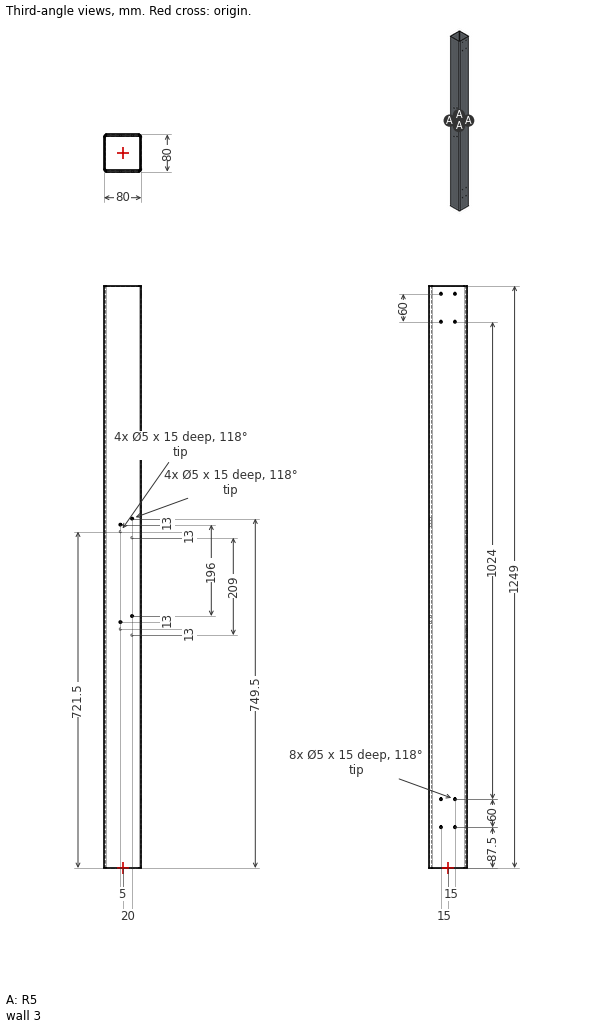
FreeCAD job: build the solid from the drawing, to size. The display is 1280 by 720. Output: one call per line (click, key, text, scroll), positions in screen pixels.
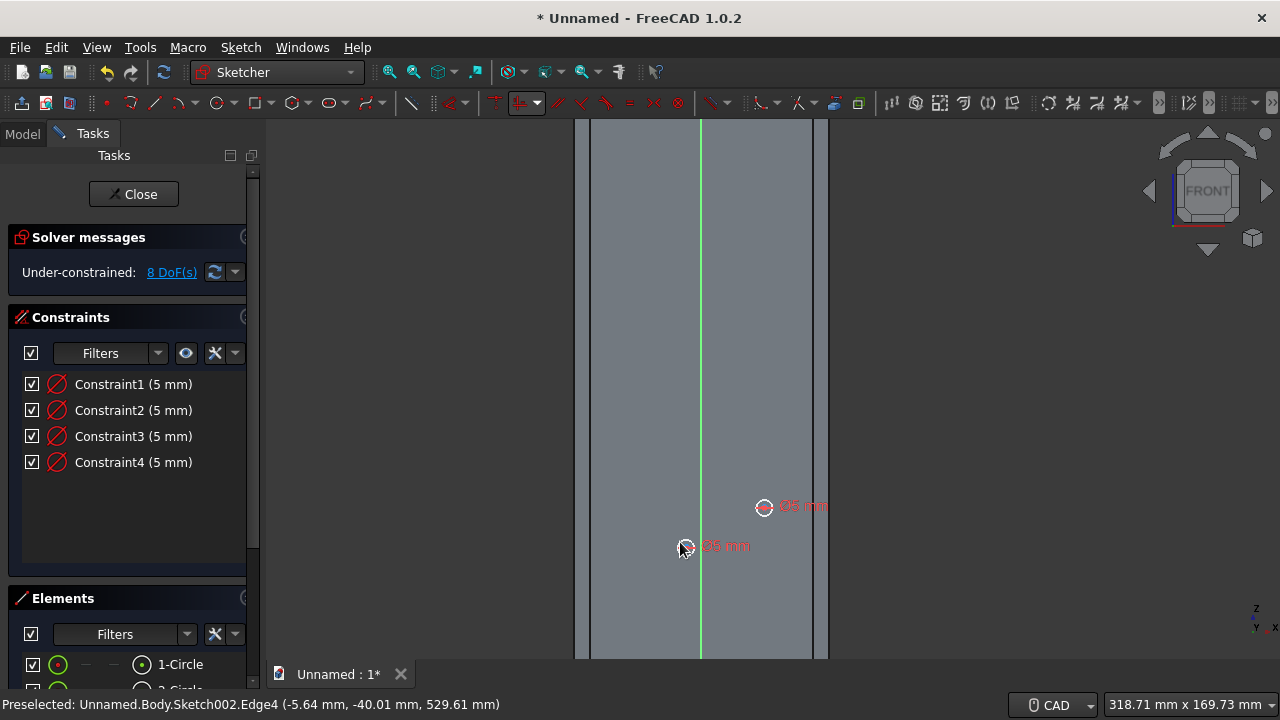
scroll(687, 548, down, 4)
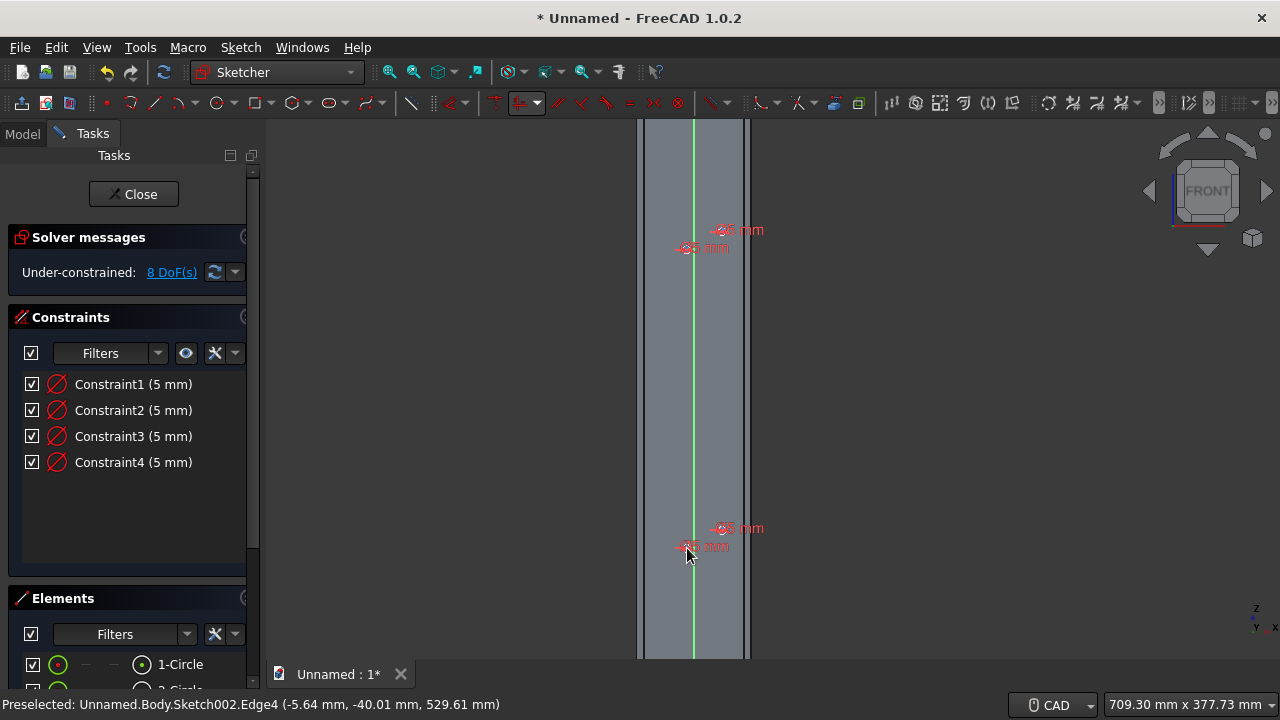
click(722, 232)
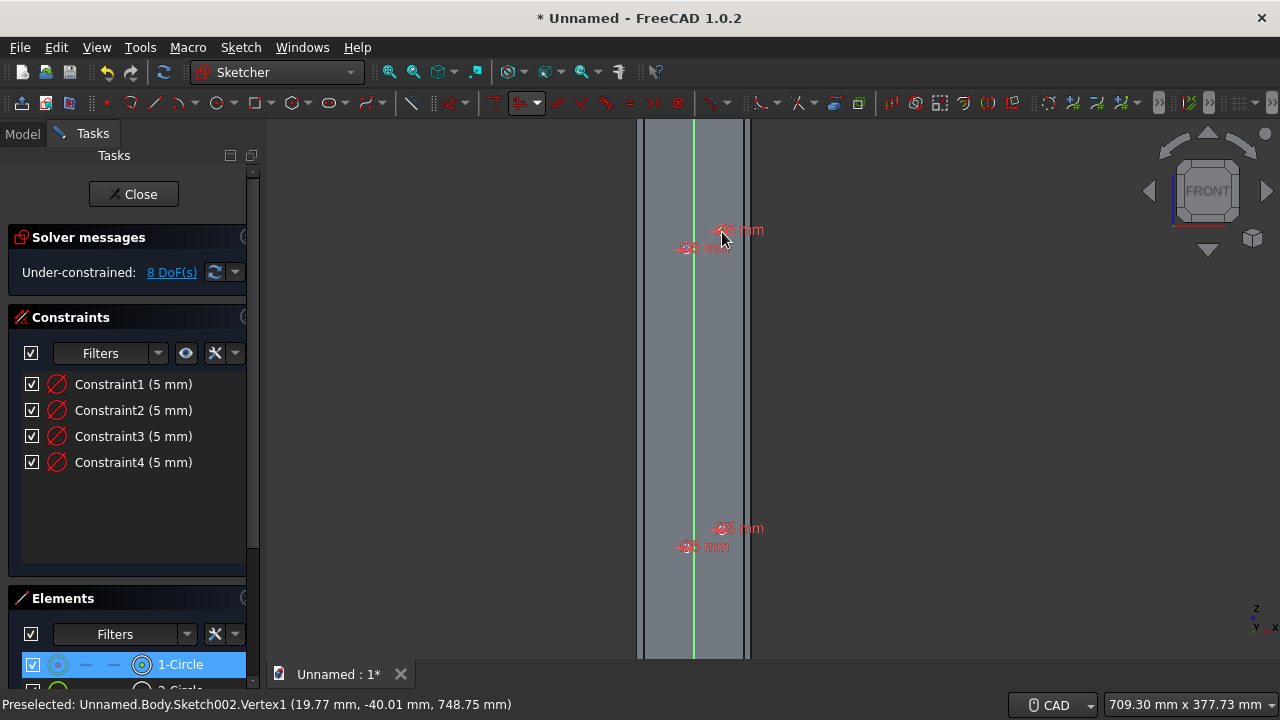
click(722, 530)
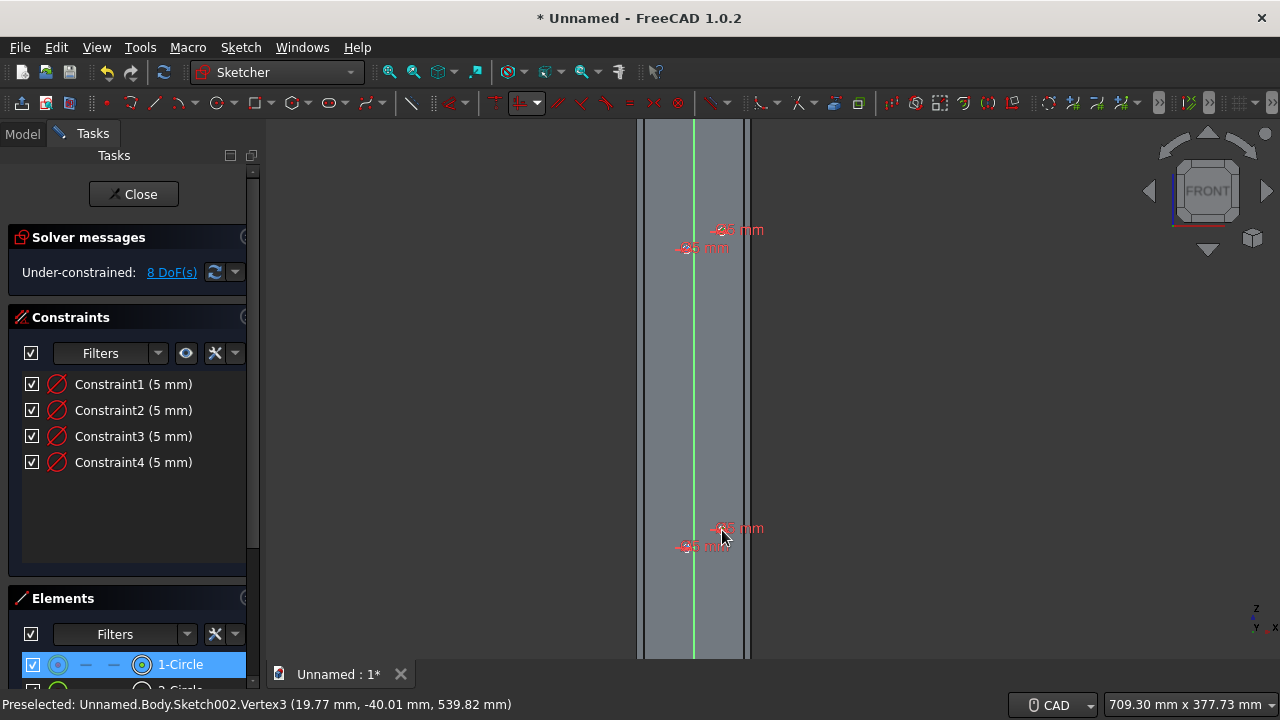
key(v)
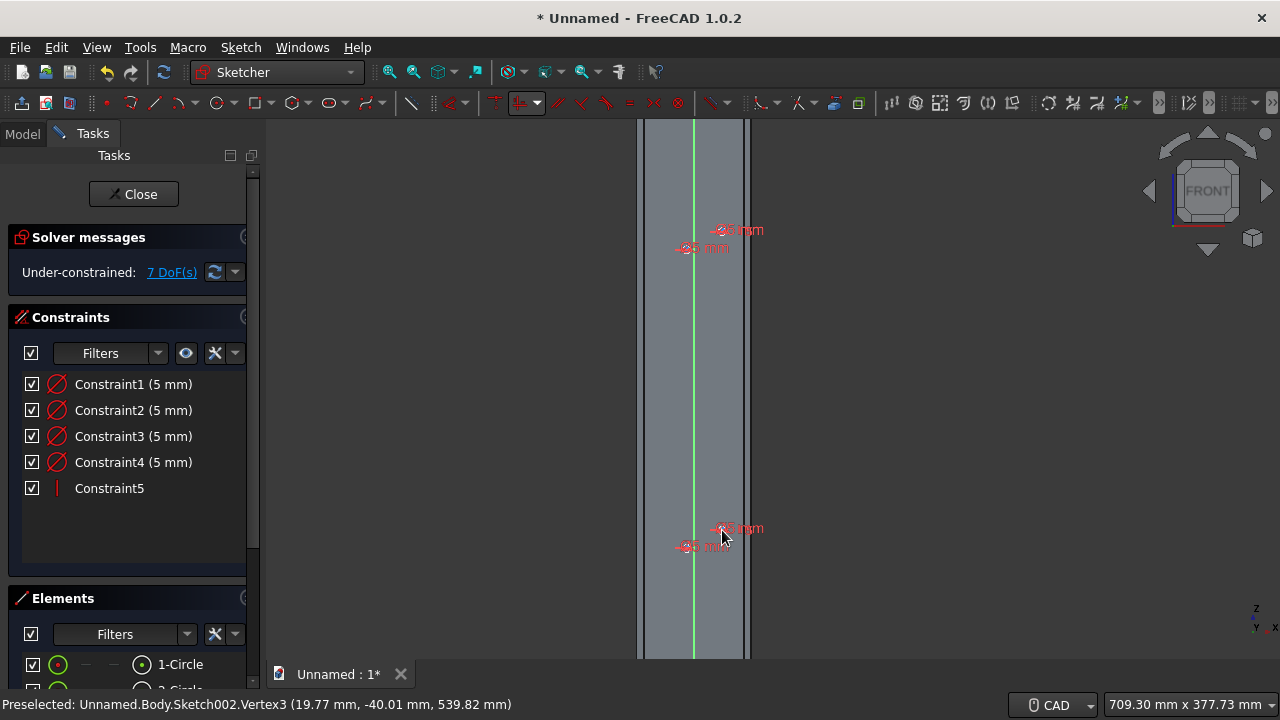
click(687, 250)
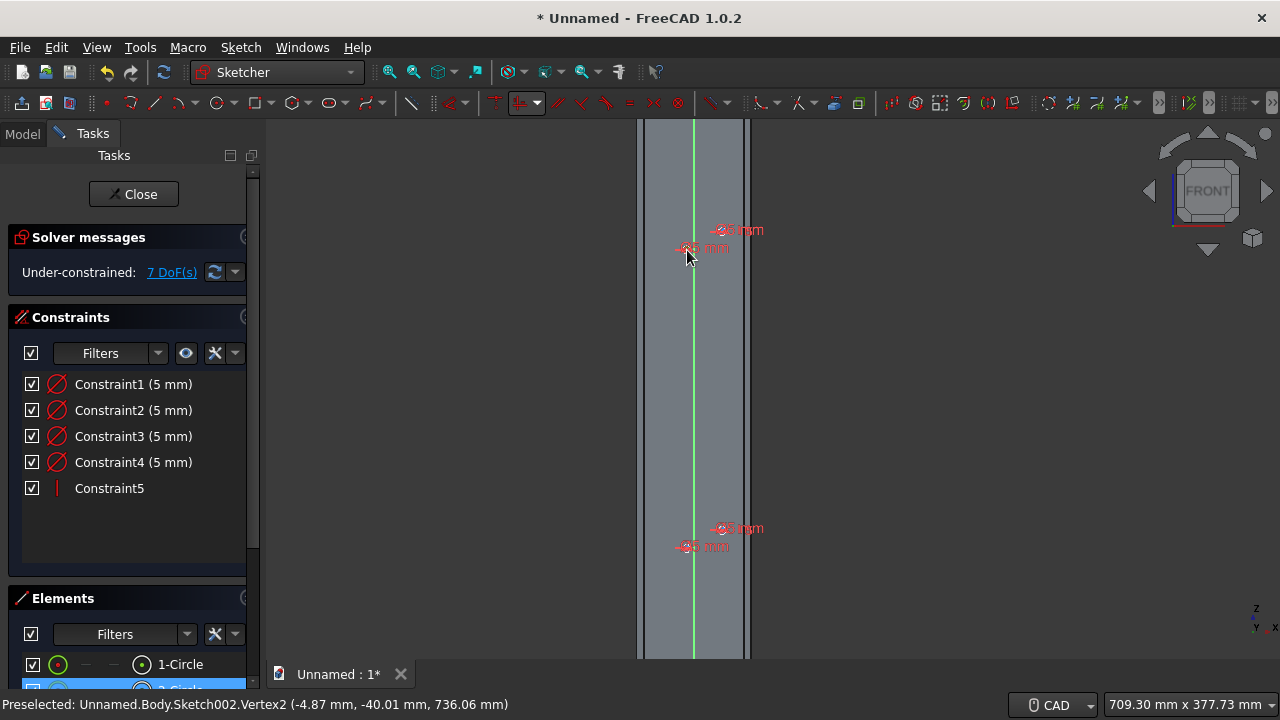
click(687, 548)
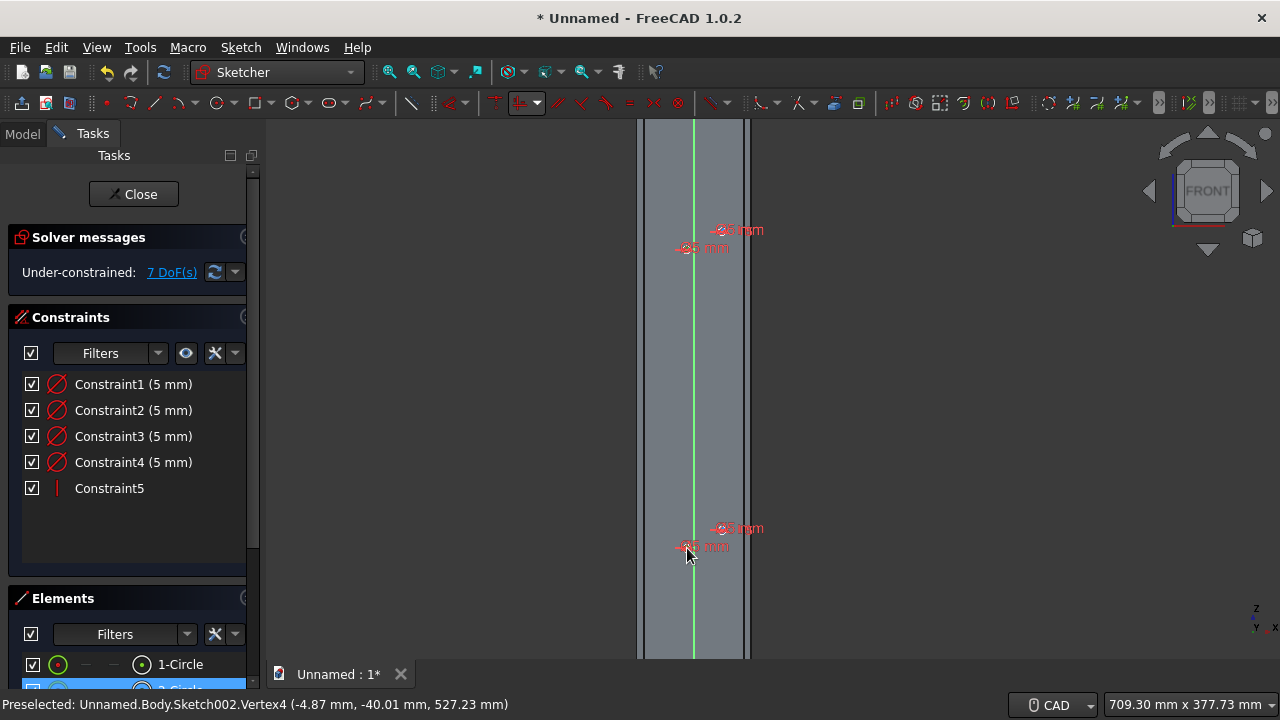
key(v)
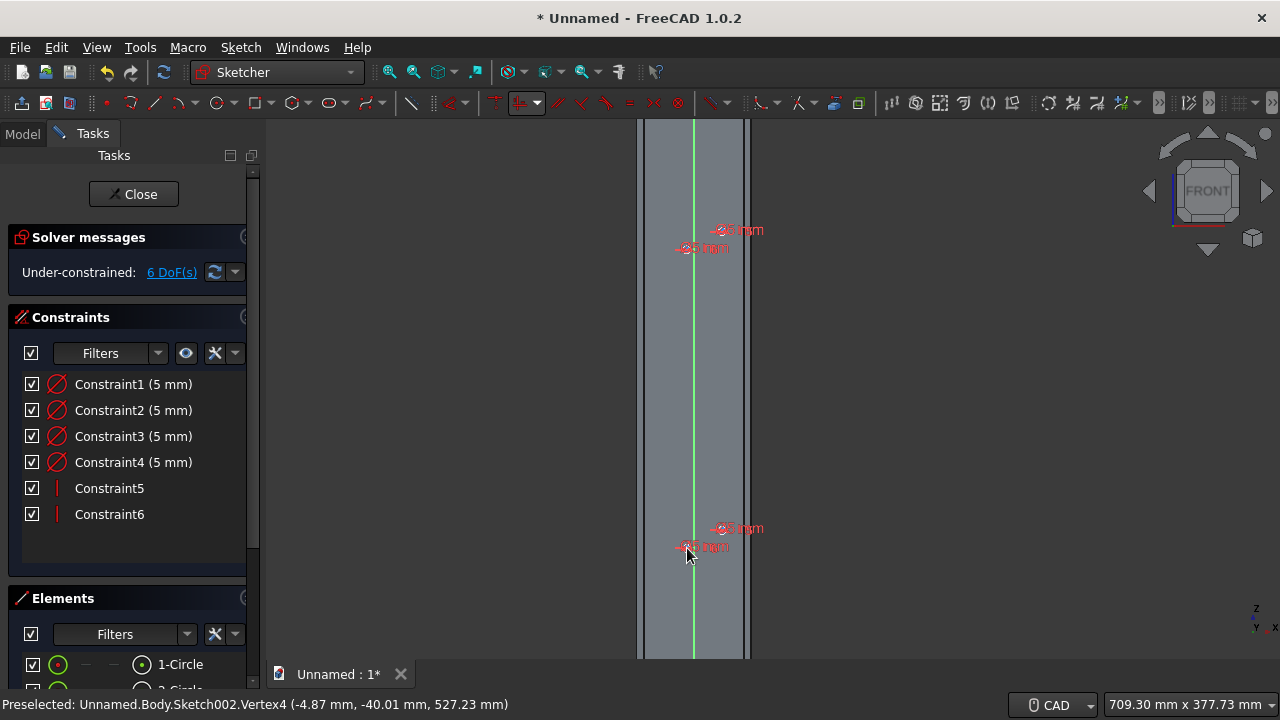
key(d)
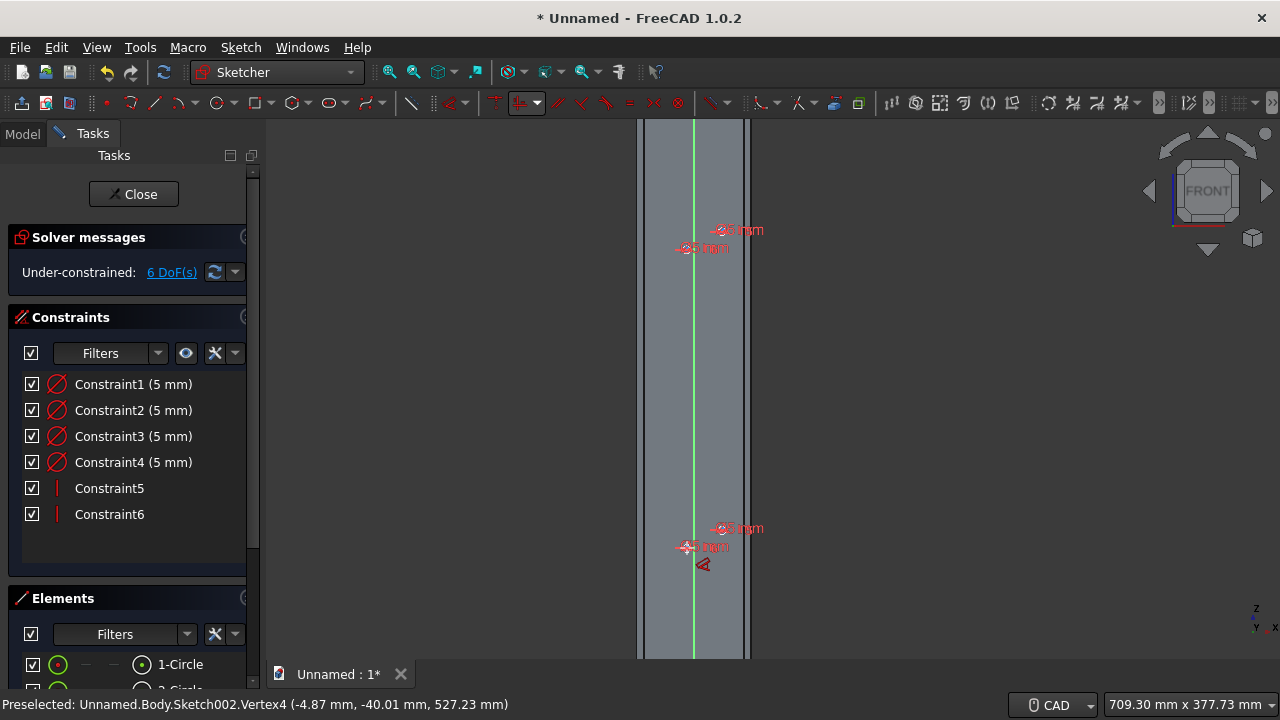
scroll(687, 250, up, 9)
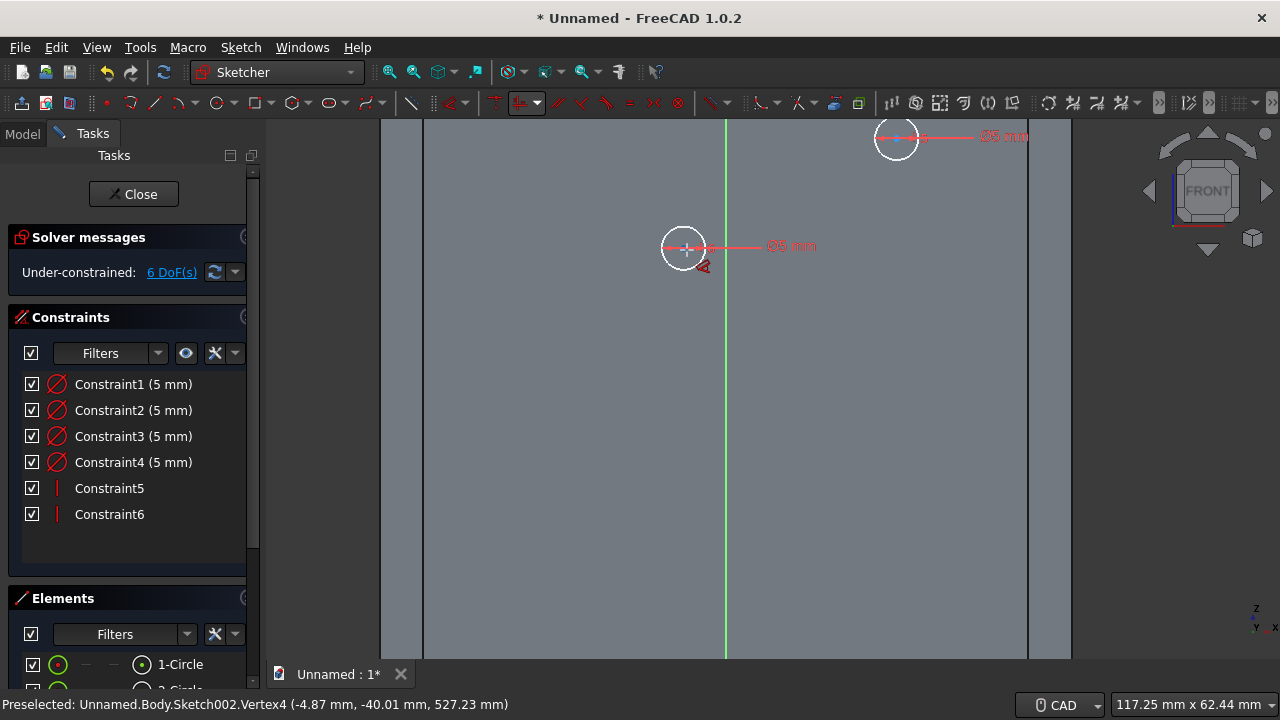
click(684, 248)
click(705, 214)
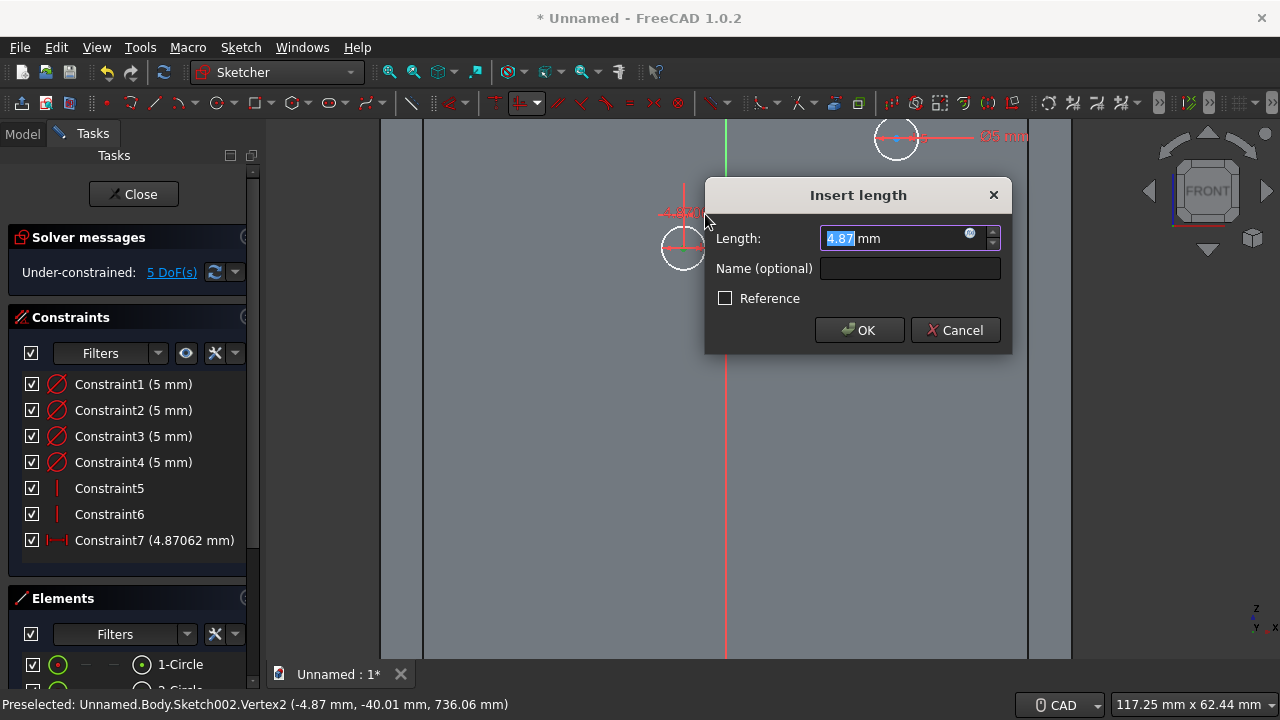
text(5)
key(Return)